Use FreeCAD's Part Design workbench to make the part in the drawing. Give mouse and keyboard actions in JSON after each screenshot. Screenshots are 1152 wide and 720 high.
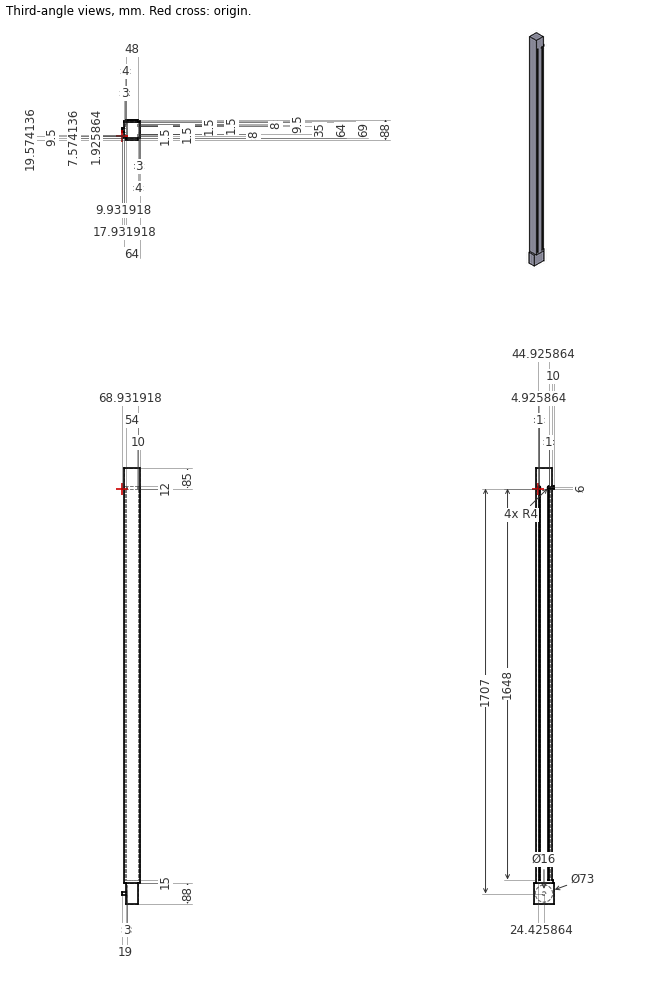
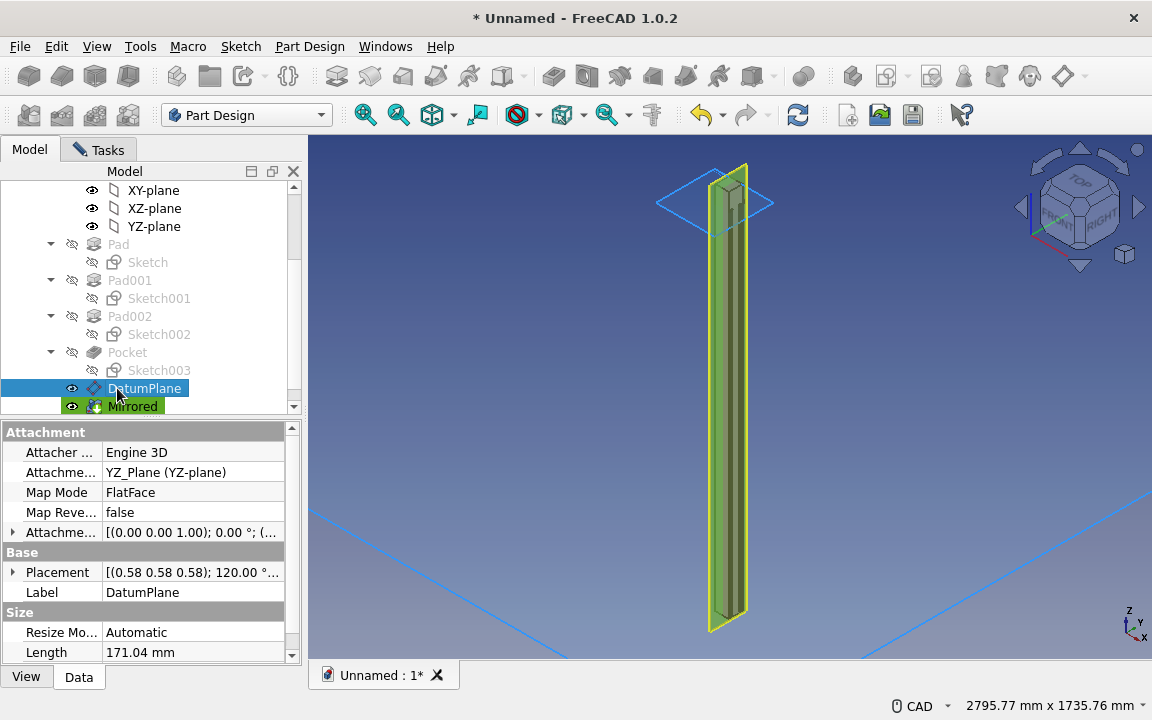
{"action": "left_click", "coordinate": [98, 149]}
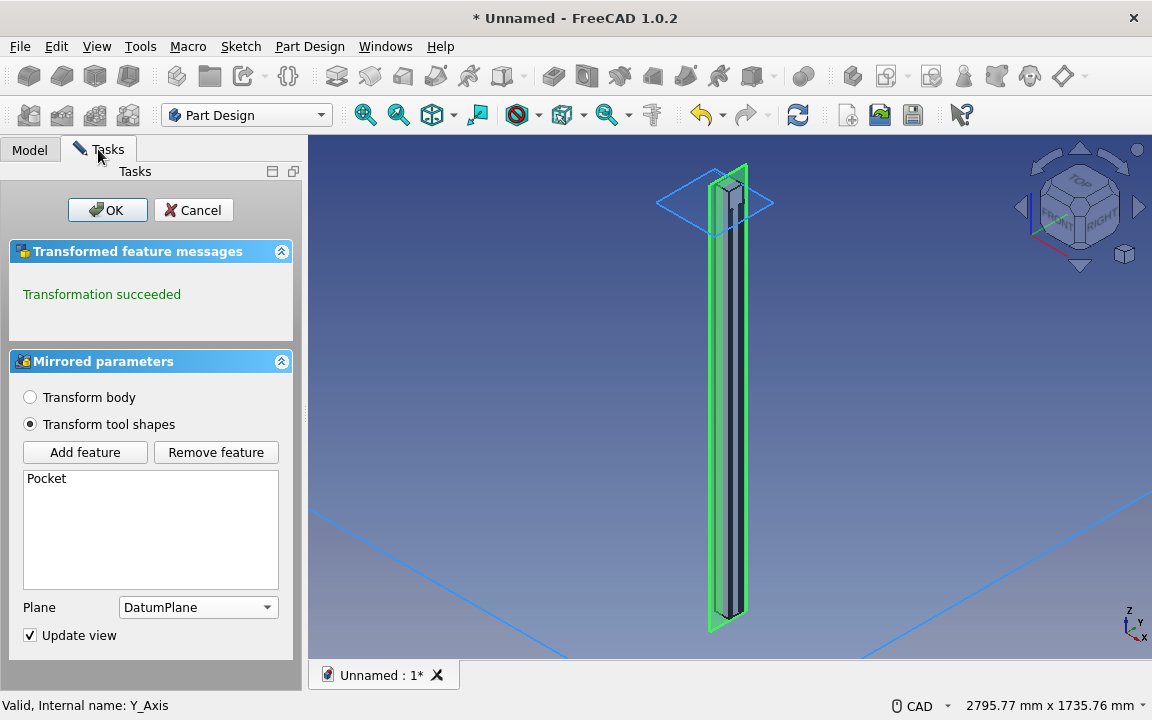
{"action": "left_click", "coordinate": [108, 210]}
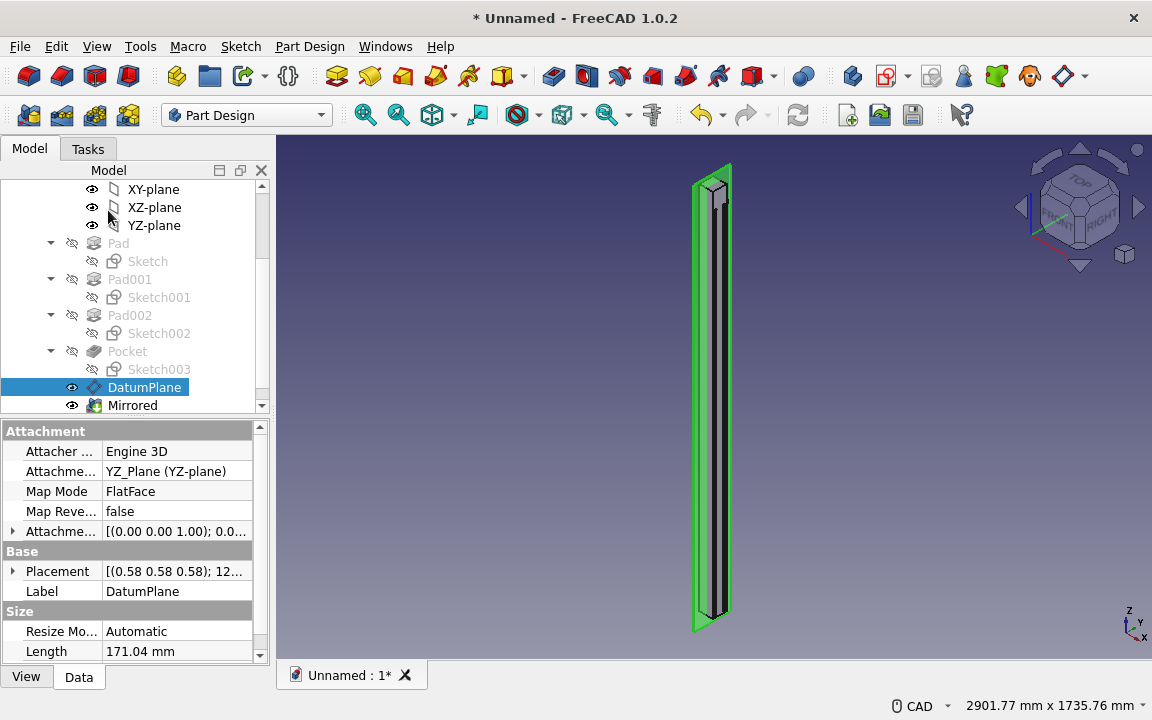
{"action": "left_click", "coordinate": [117, 387]}
{"action": "key", "text": "space"}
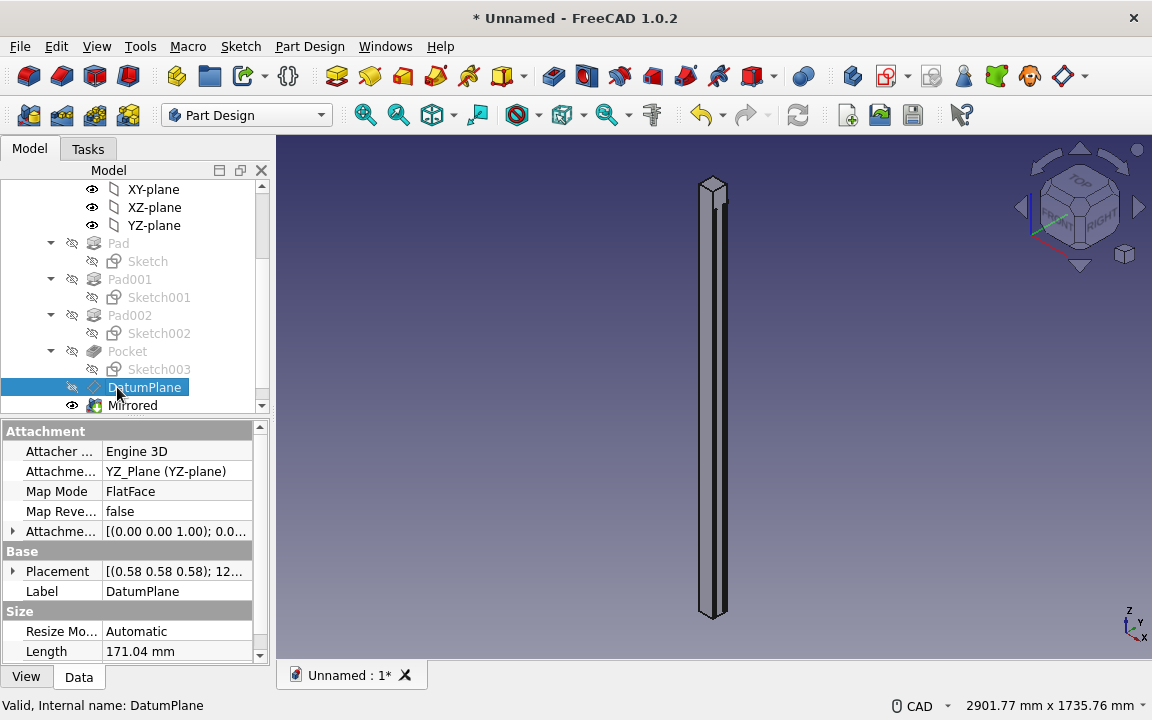
{"action": "key", "text": "5"}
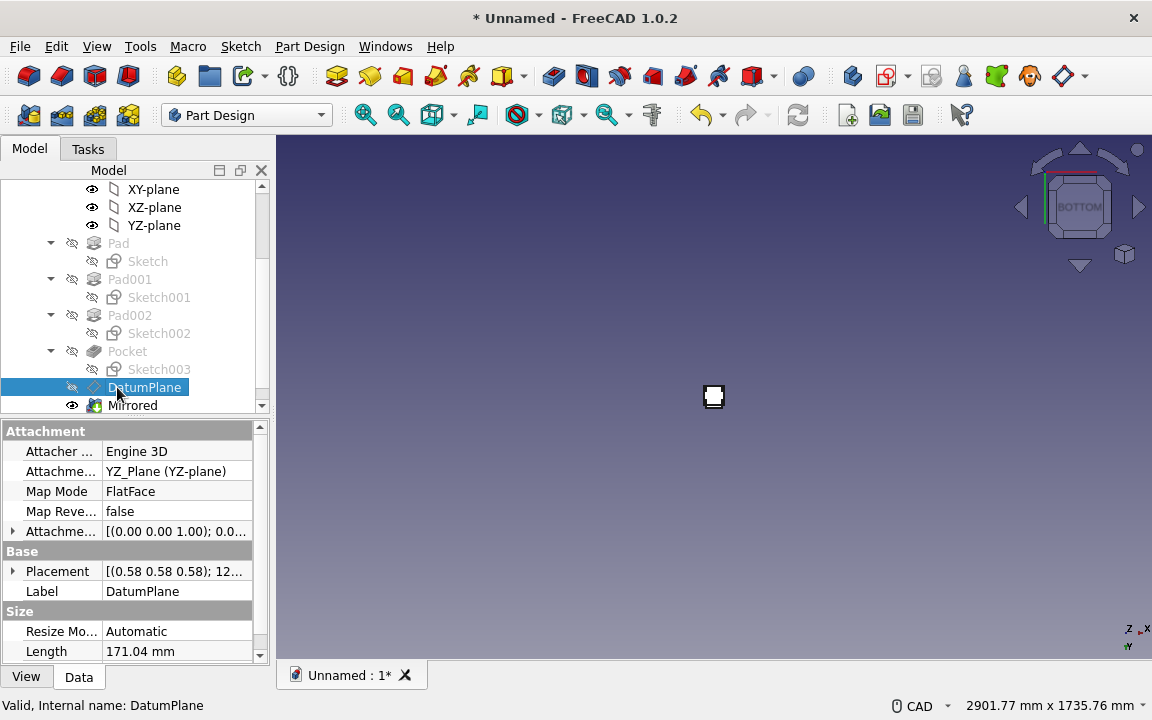
{"action": "left_click", "coordinate": [366, 116]}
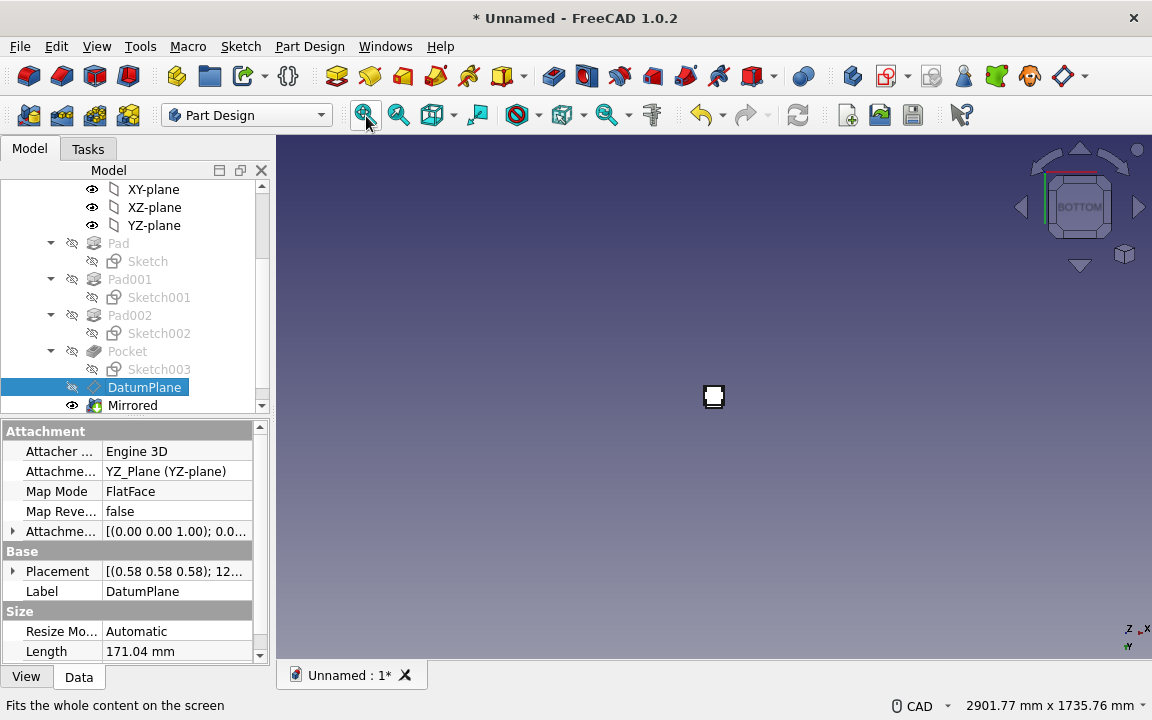
{"action": "key", "text": "1"}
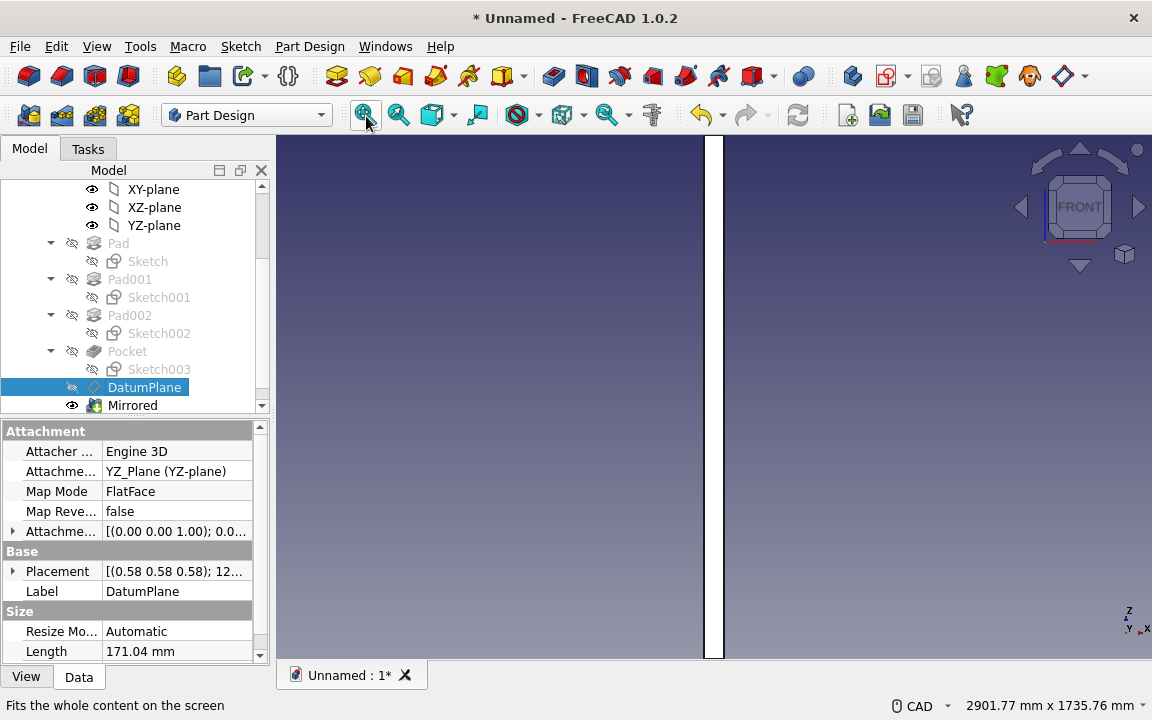
{"action": "left_click", "coordinate": [366, 116]}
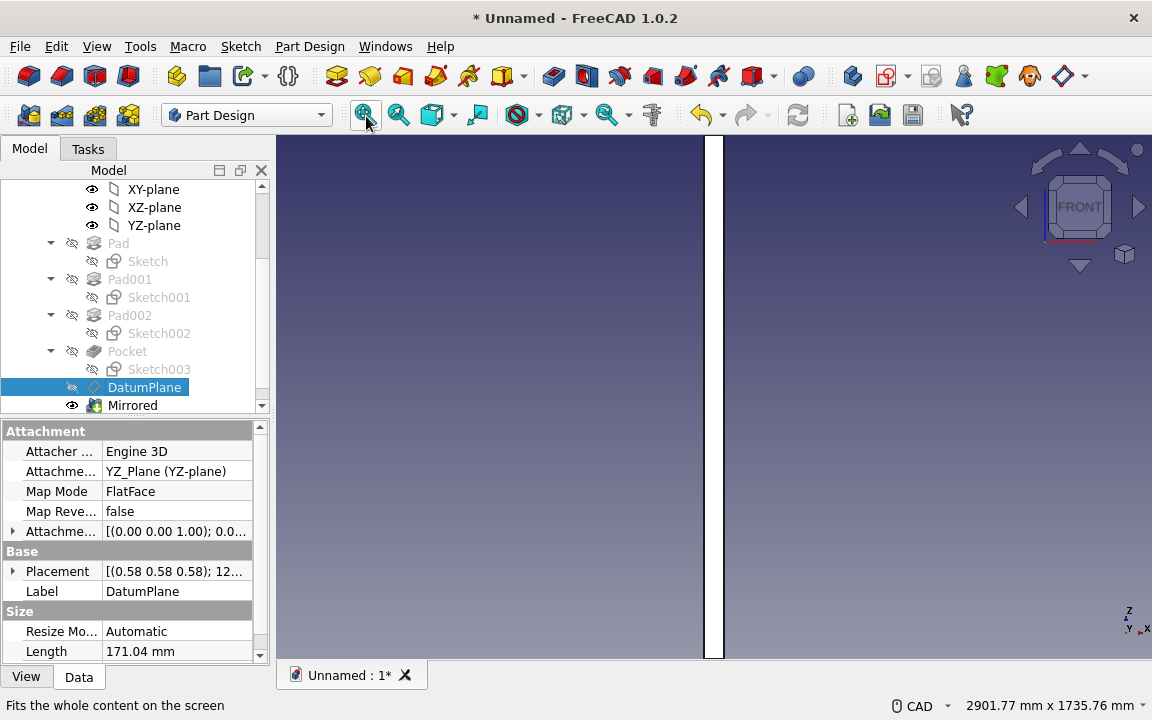
{"action": "key", "text": "3"}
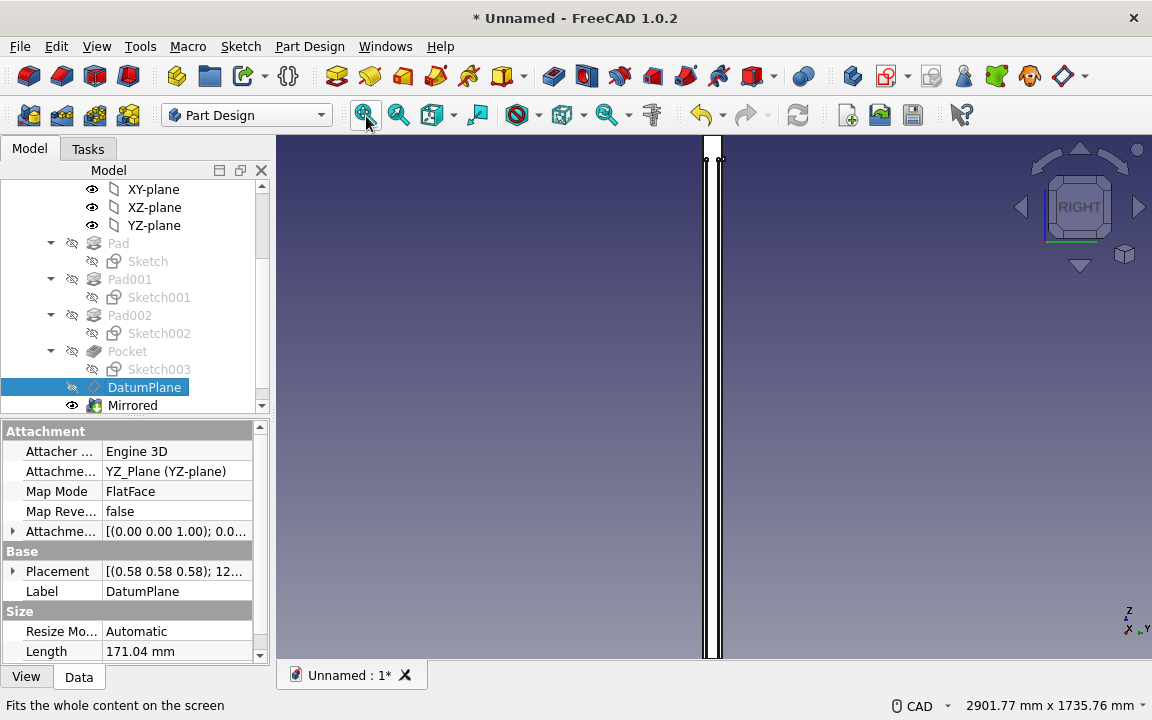
{"action": "left_click", "coordinate": [366, 116]}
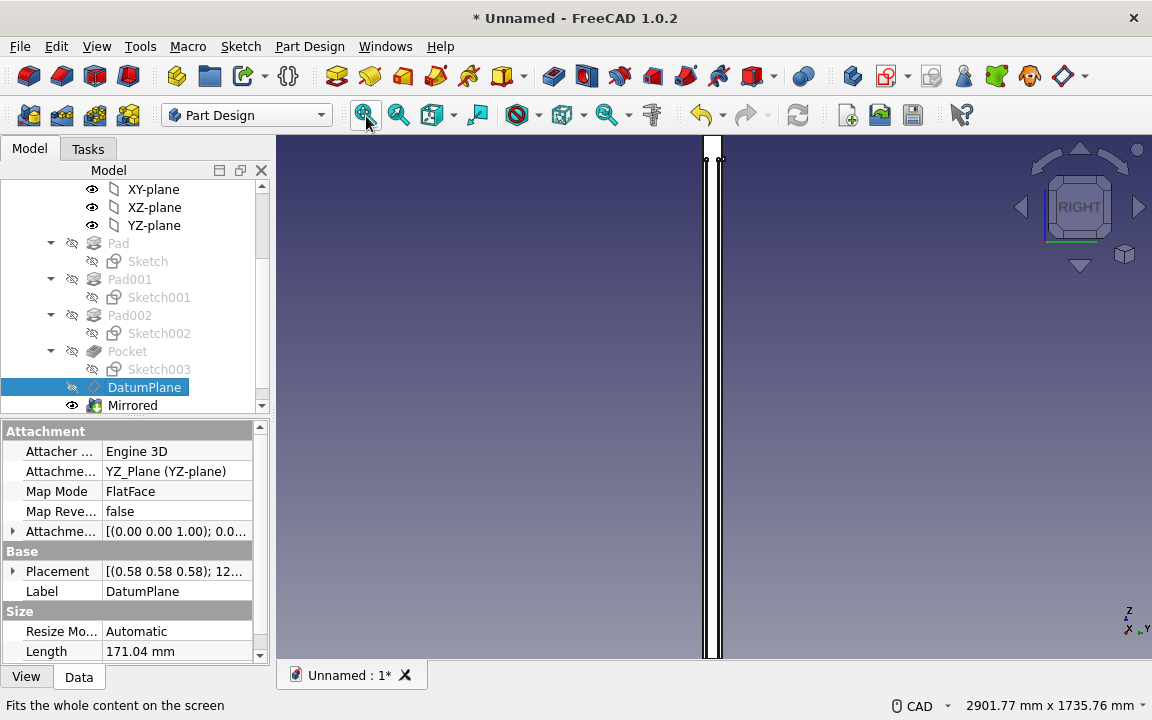
{"action": "scroll", "coordinate": [161, 293], "scroll_direction": "down", "scroll_amount": 3}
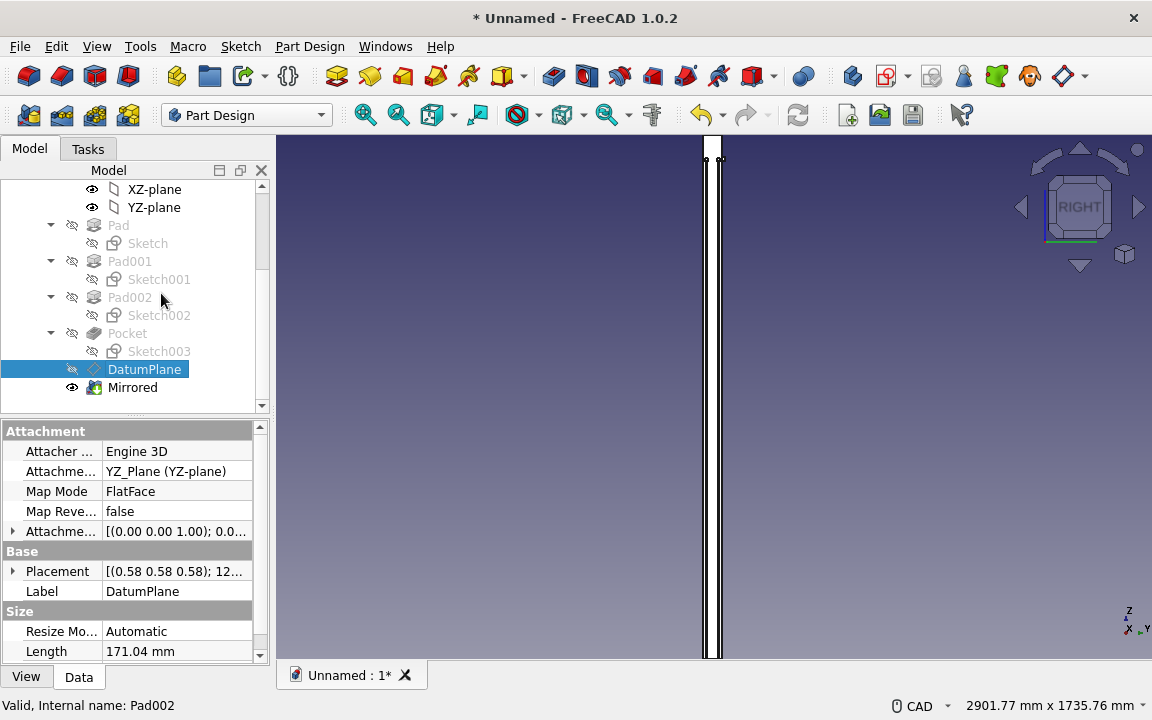
{"action": "scroll", "coordinate": [161, 293], "scroll_direction": "up", "scroll_amount": 15}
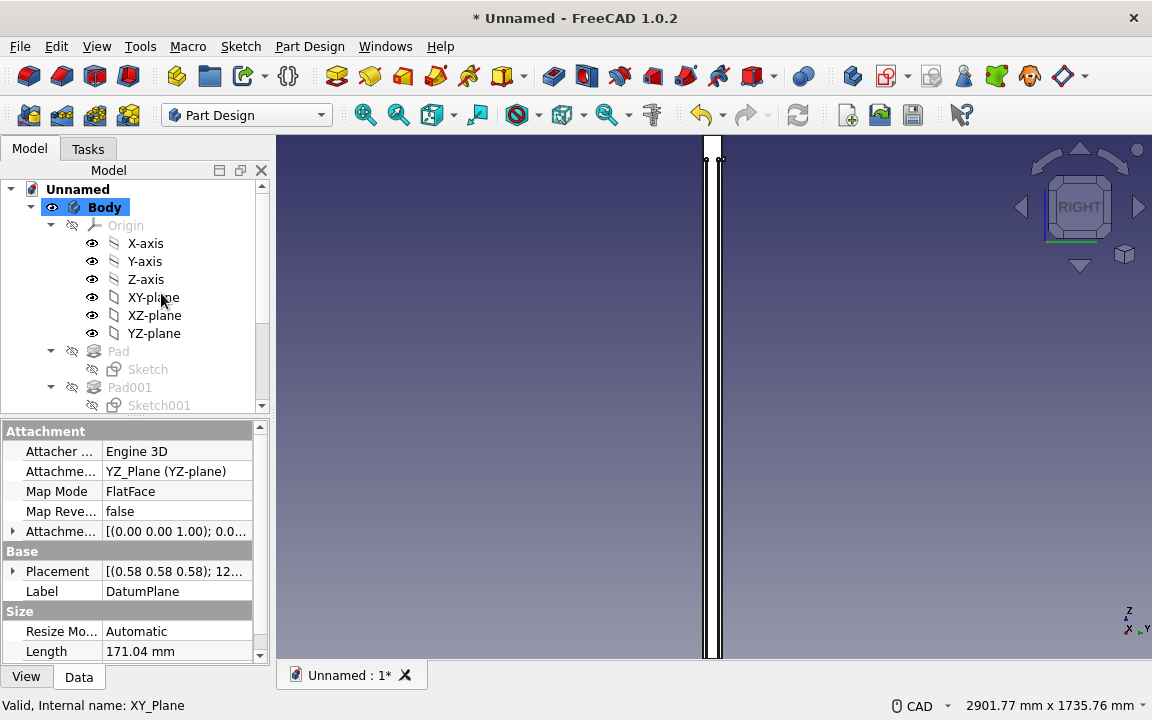
{"action": "left_click", "coordinate": [137, 297]}